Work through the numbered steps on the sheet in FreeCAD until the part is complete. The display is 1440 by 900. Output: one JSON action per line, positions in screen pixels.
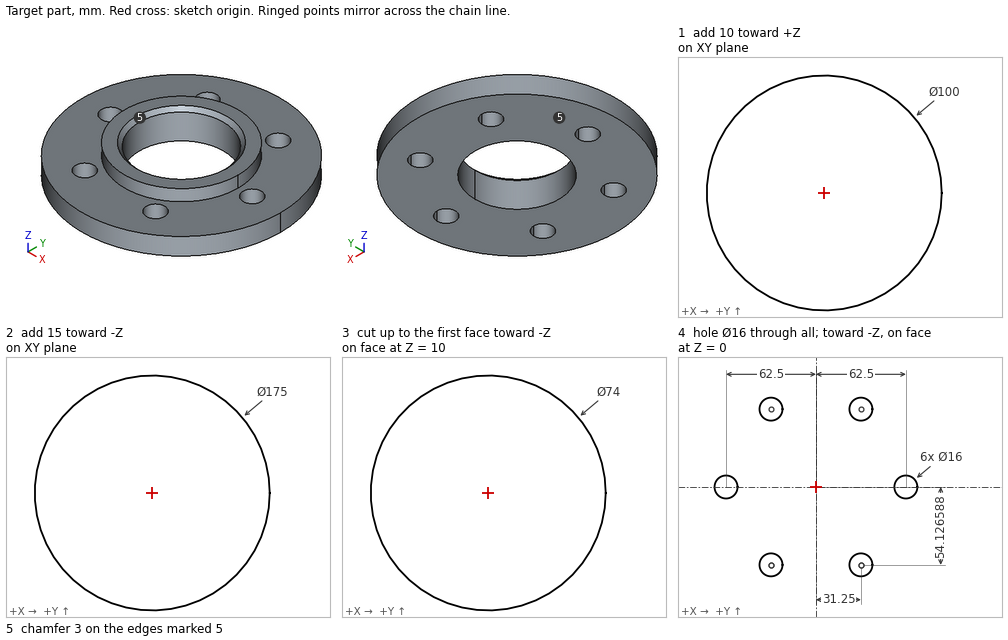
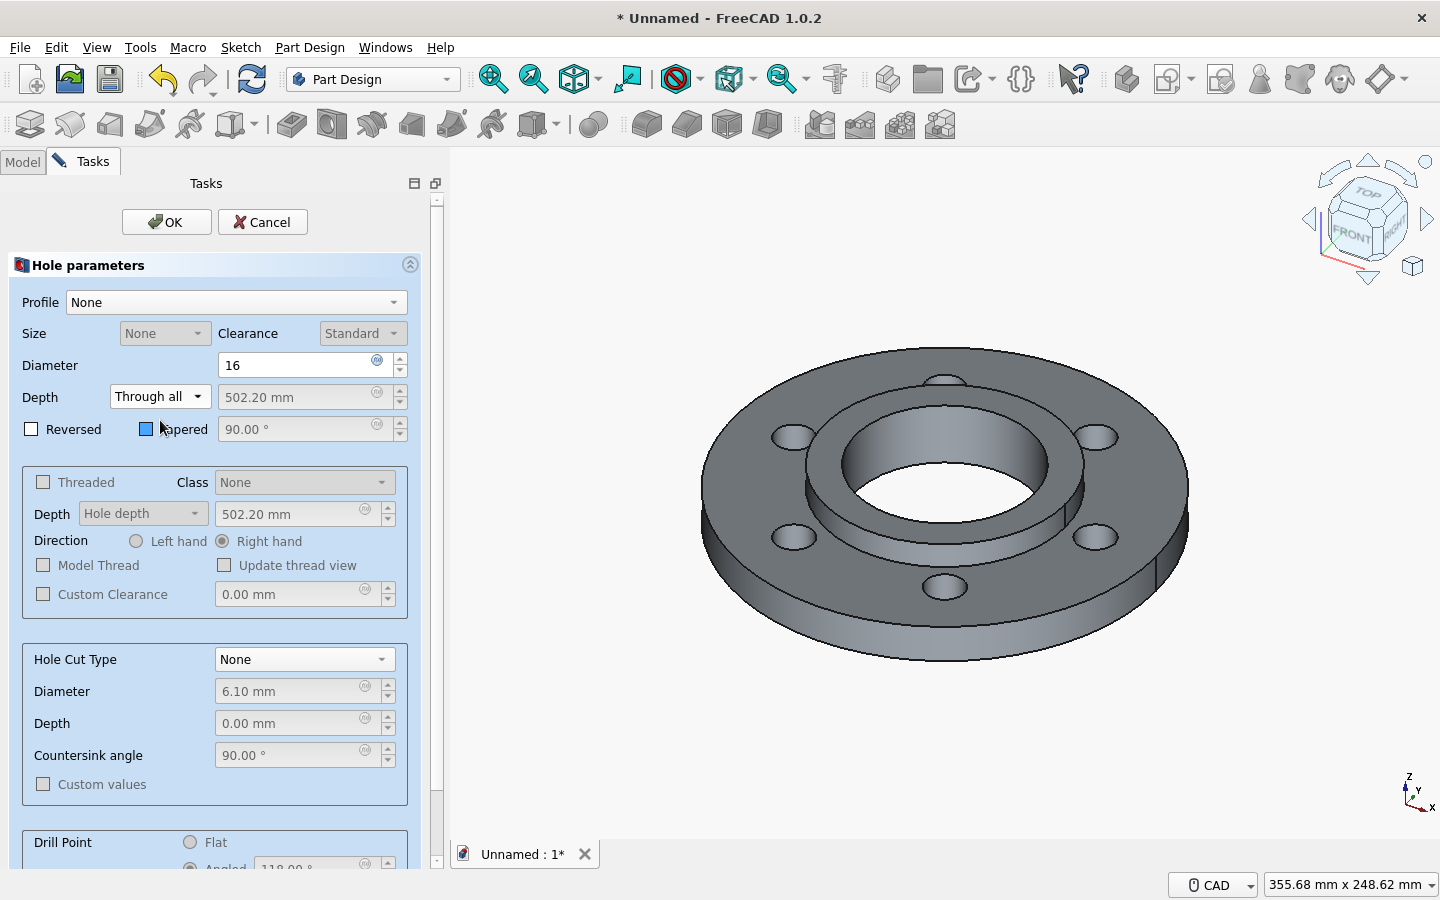
{"action": "left_click", "coordinate": [167, 222]}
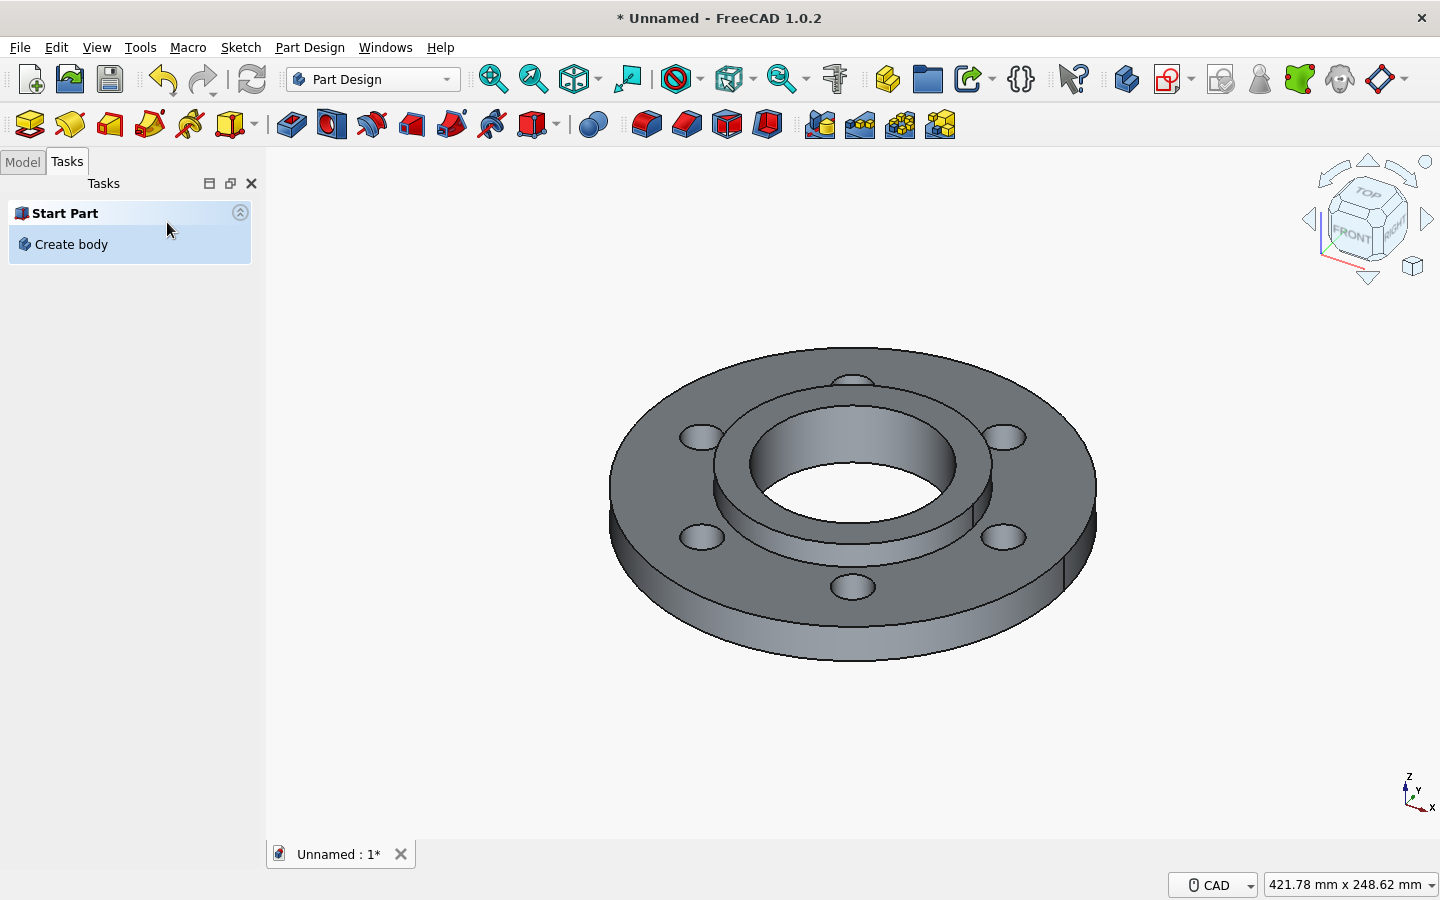
{"action": "left_click", "coordinate": [764, 434]}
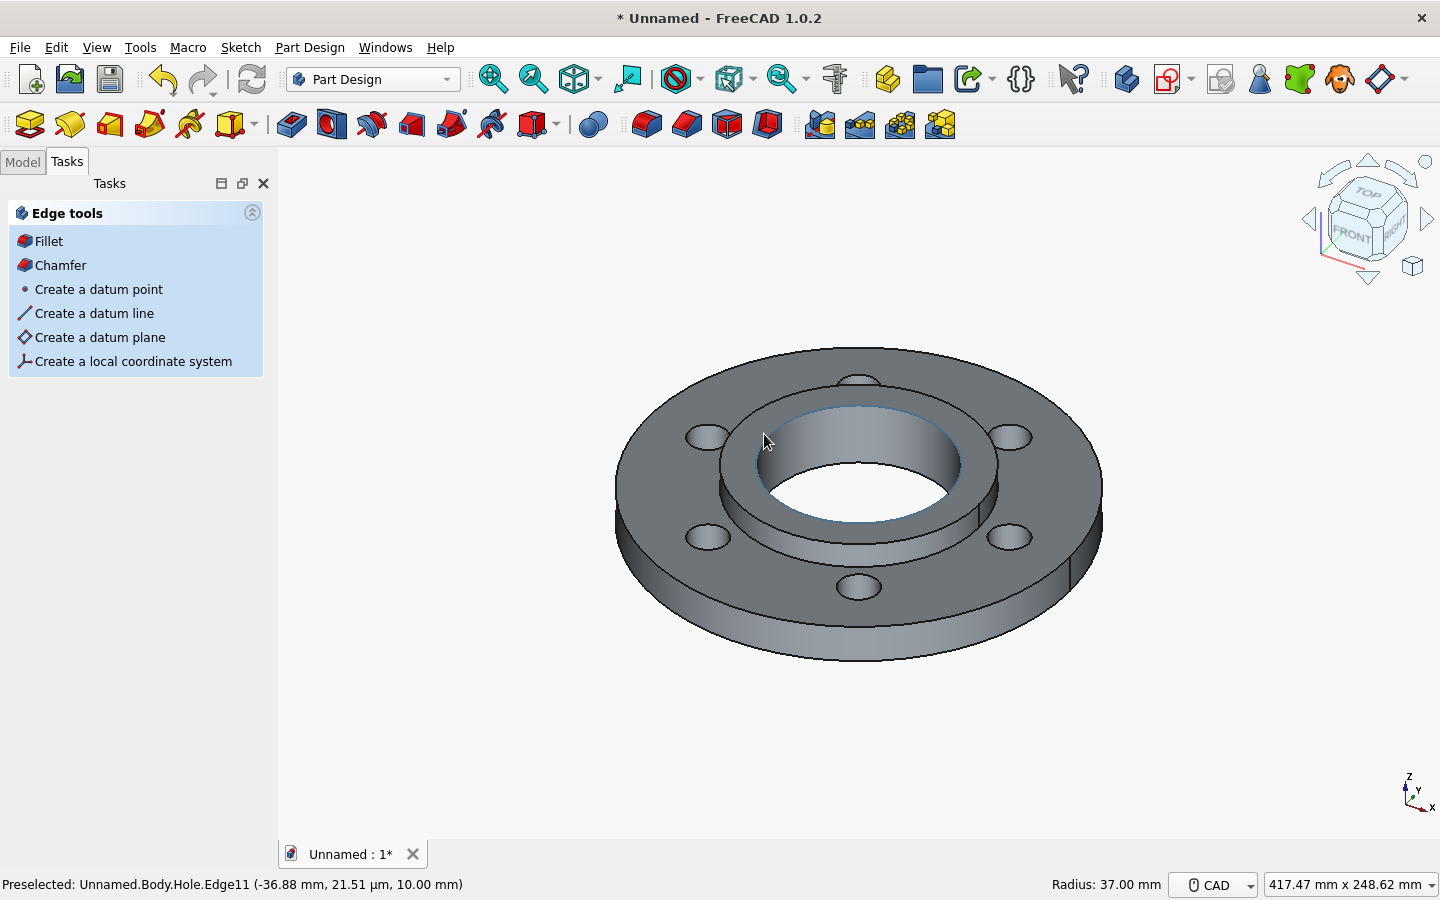
{"action": "left_click", "coordinate": [688, 124]}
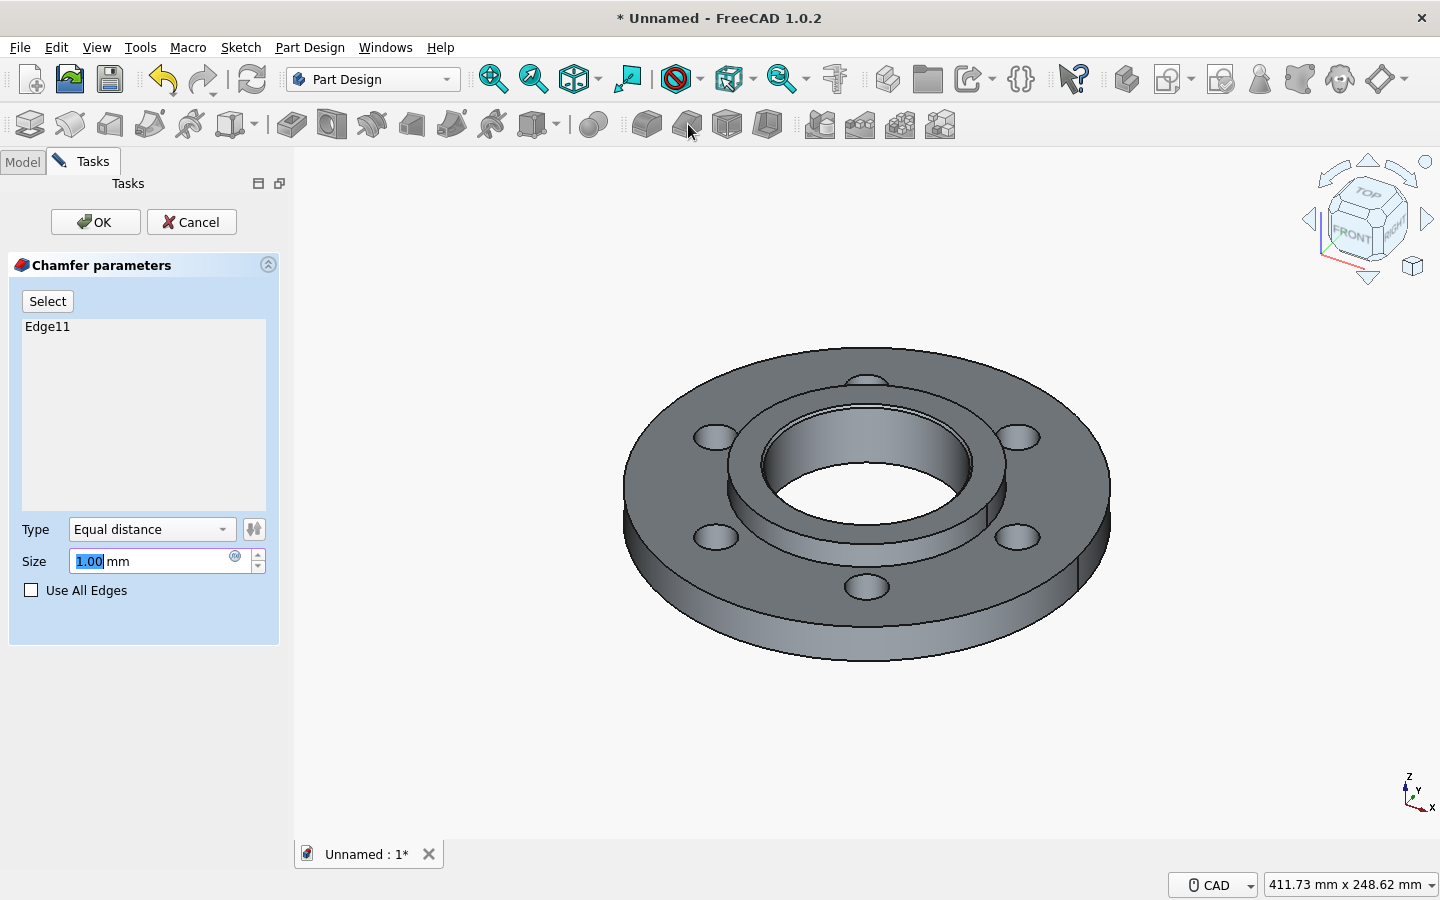
{"action": "type", "text": "3"}
{"action": "key", "text": "Tab"}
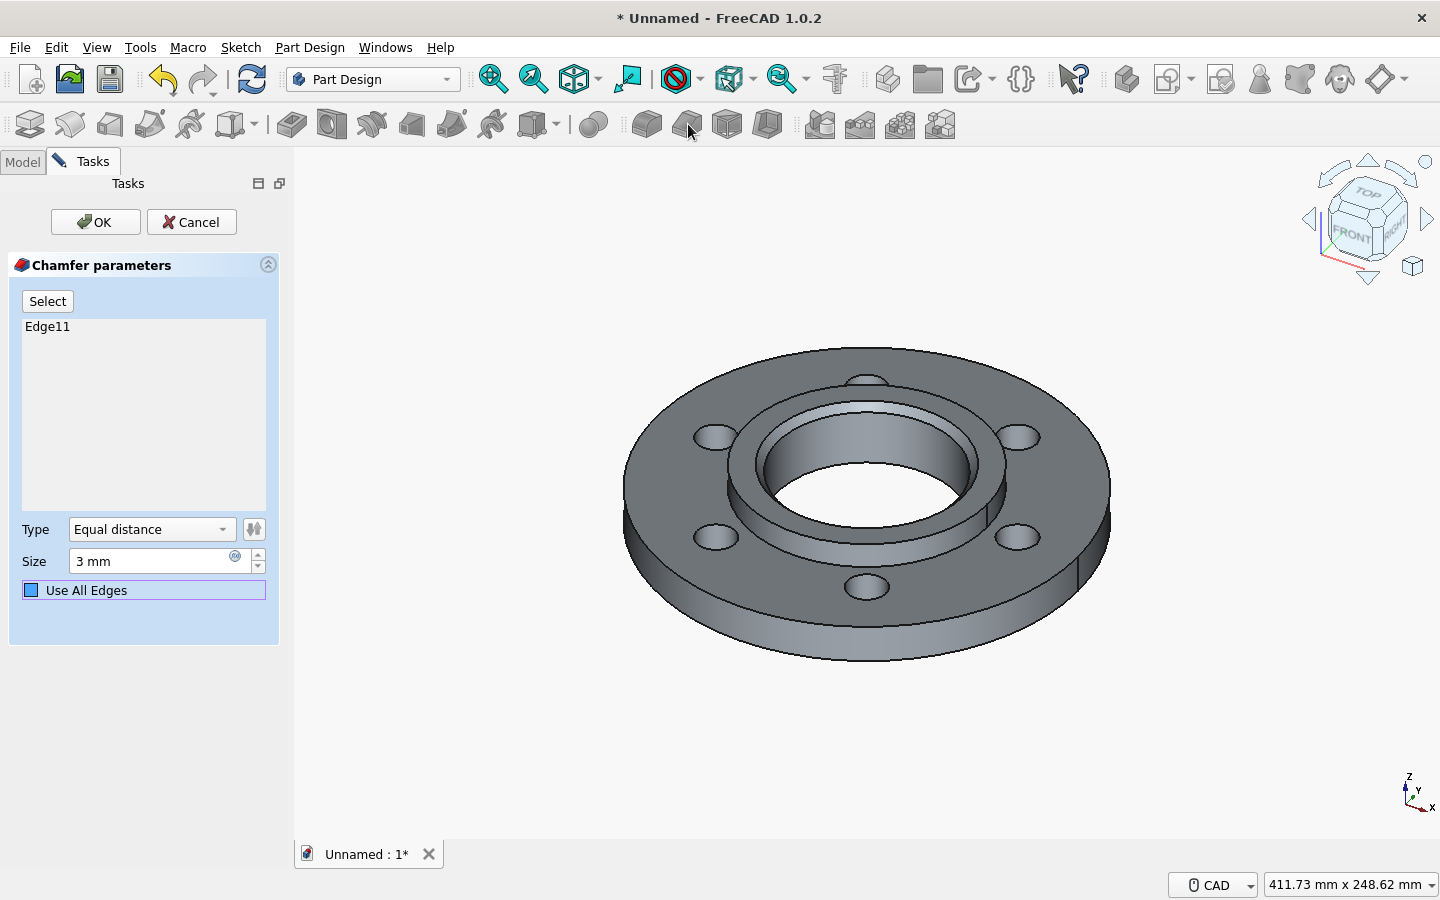
{"action": "left_click", "coordinate": [96, 222]}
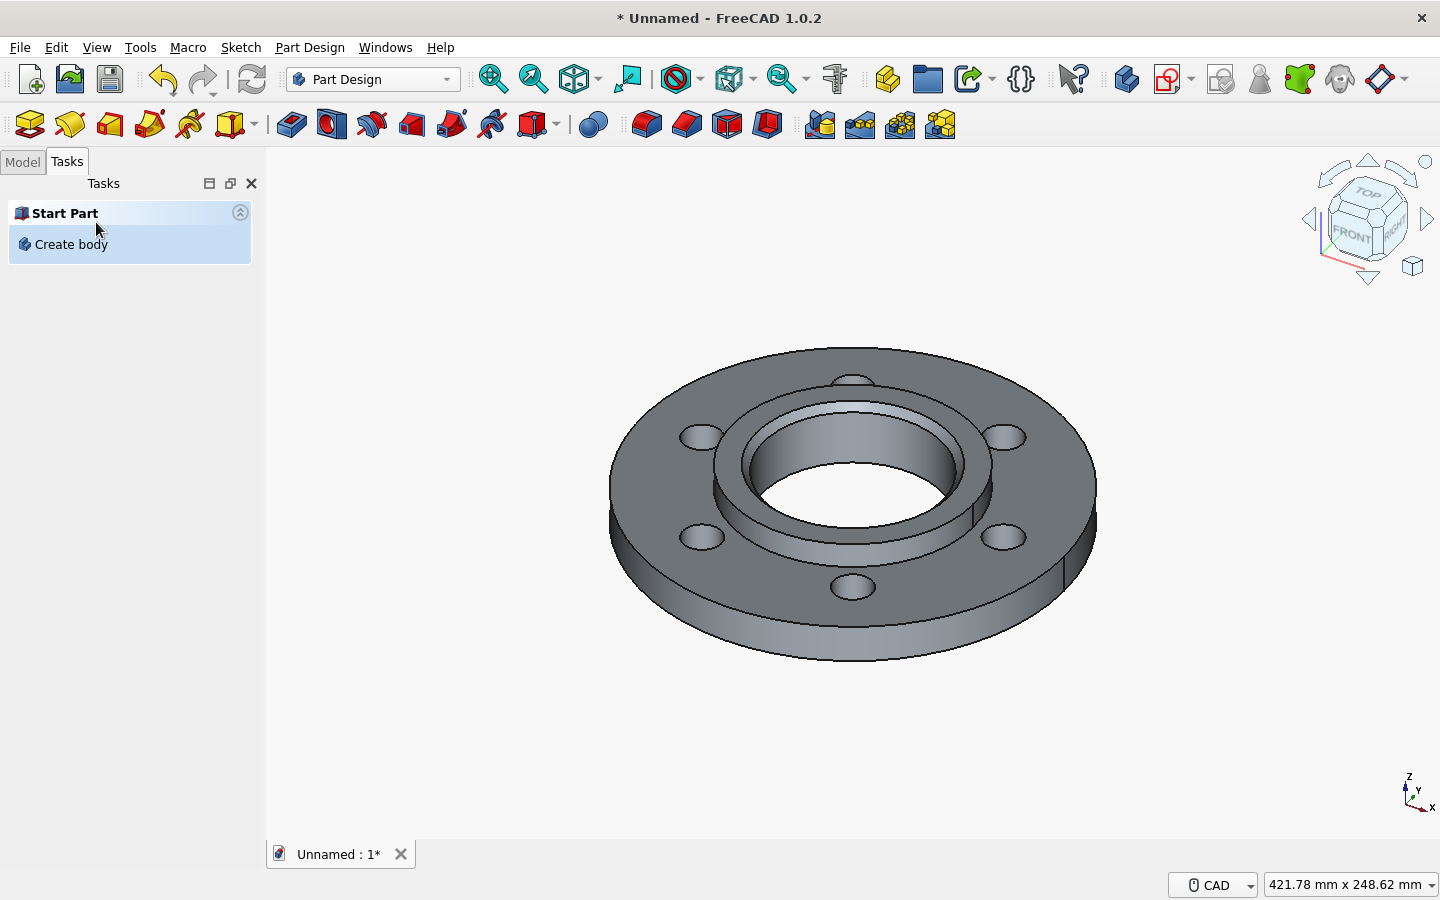
{"action": "key", "text": "0"}